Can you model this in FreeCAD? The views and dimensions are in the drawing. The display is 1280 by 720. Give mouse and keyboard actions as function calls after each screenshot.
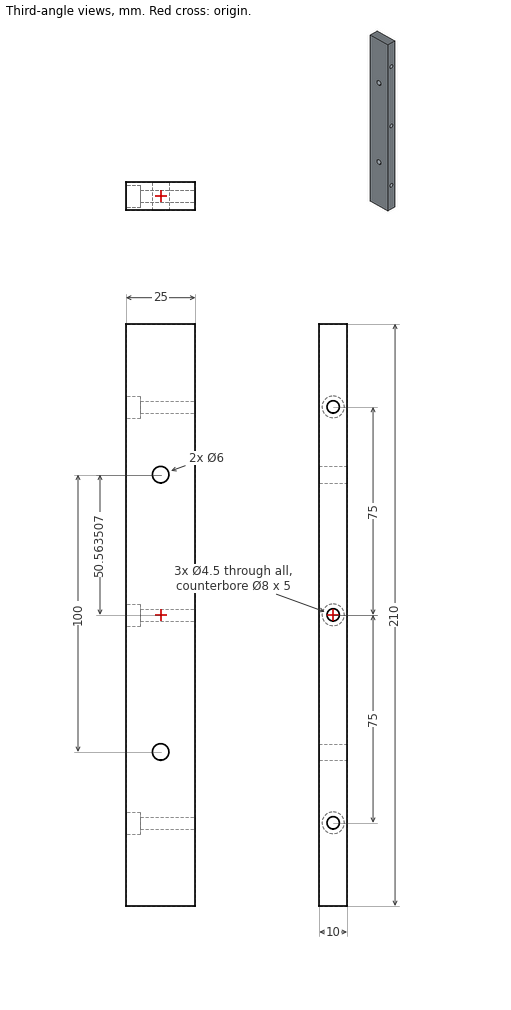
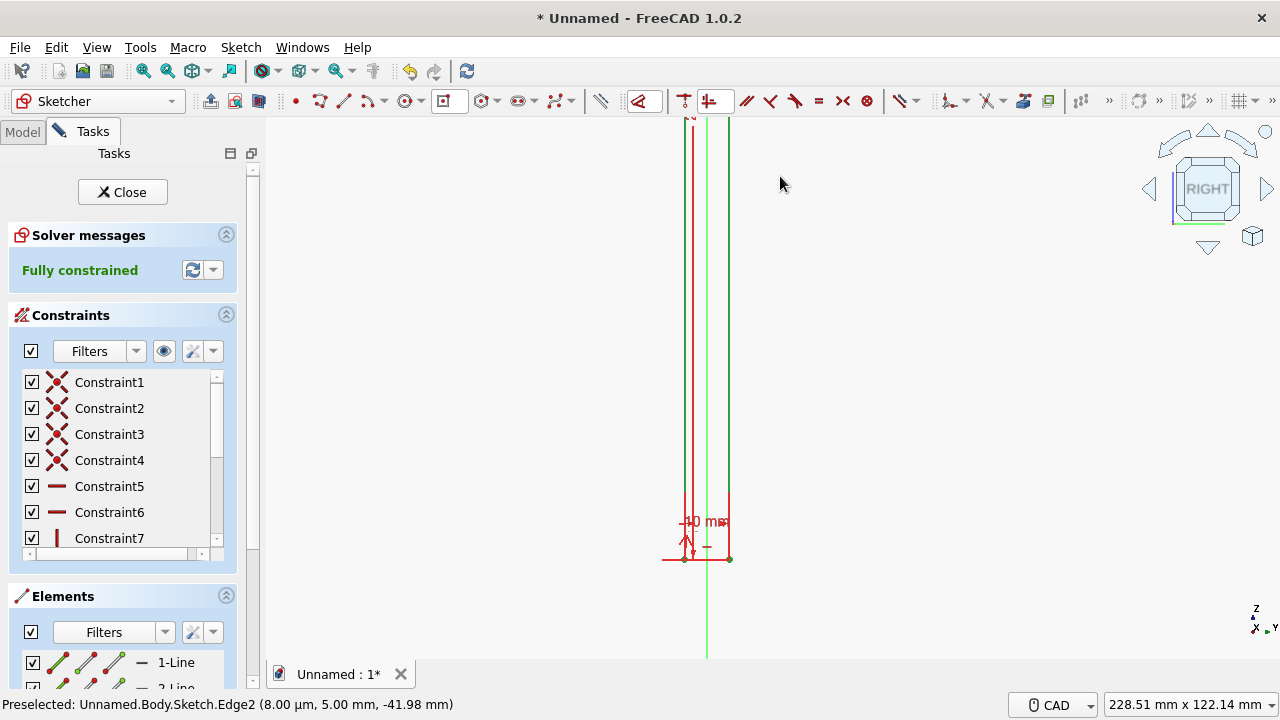
click(123, 192)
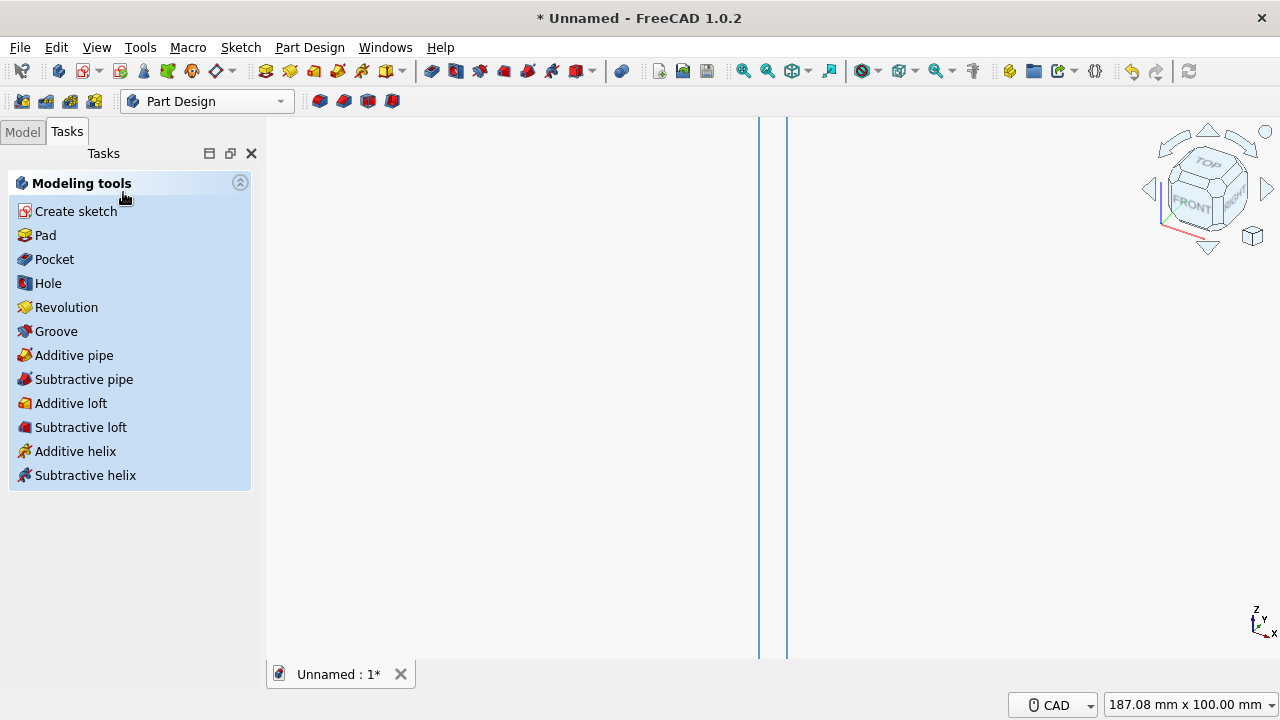
click(266, 72)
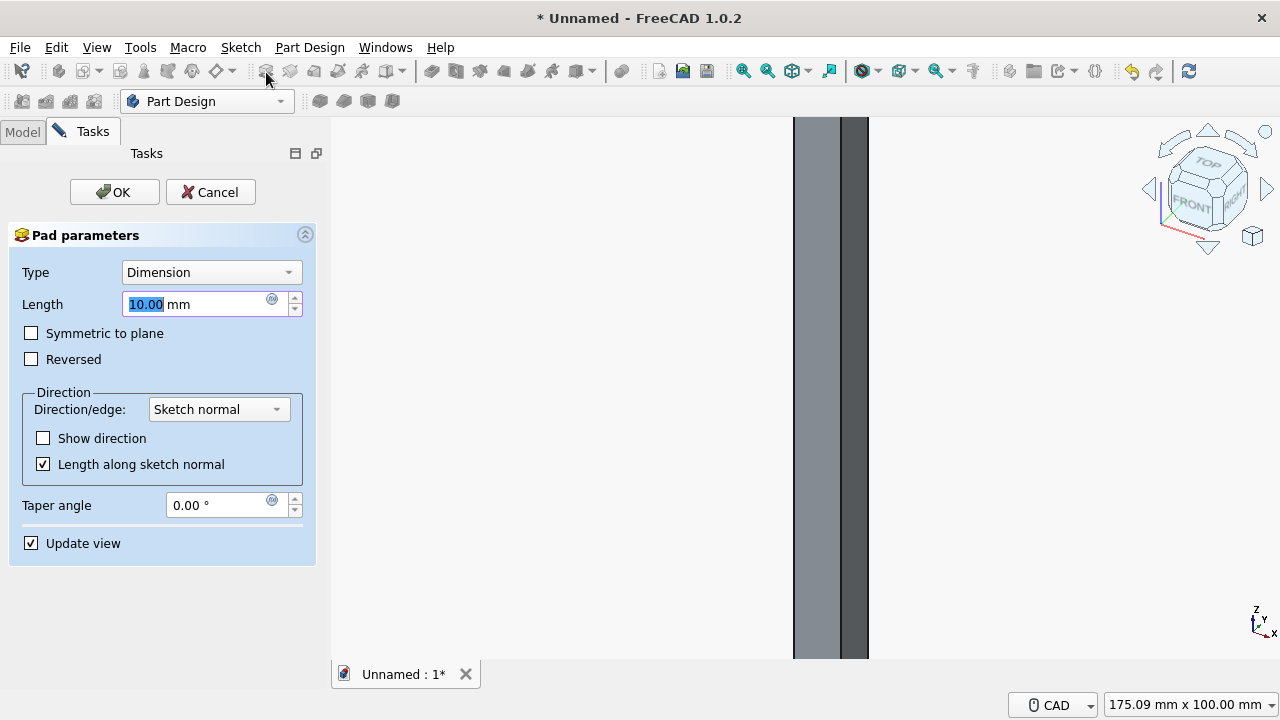
text(25)
key(Tab)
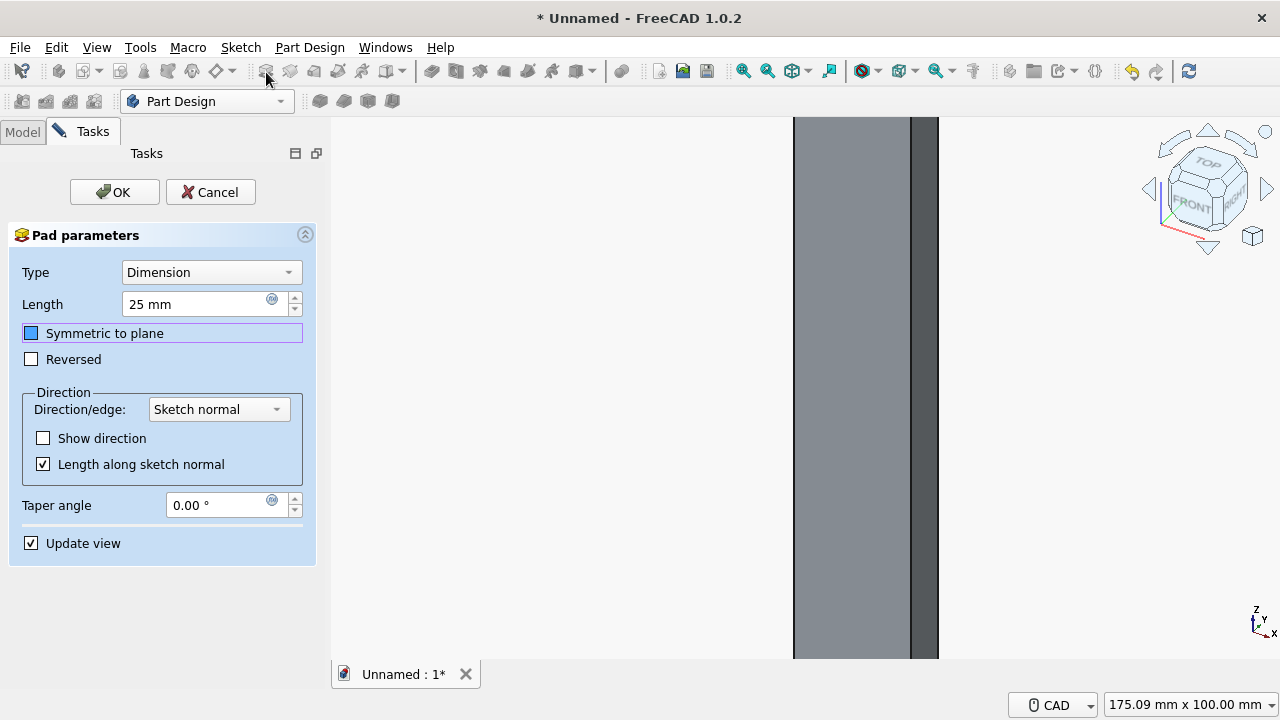
click(30, 333)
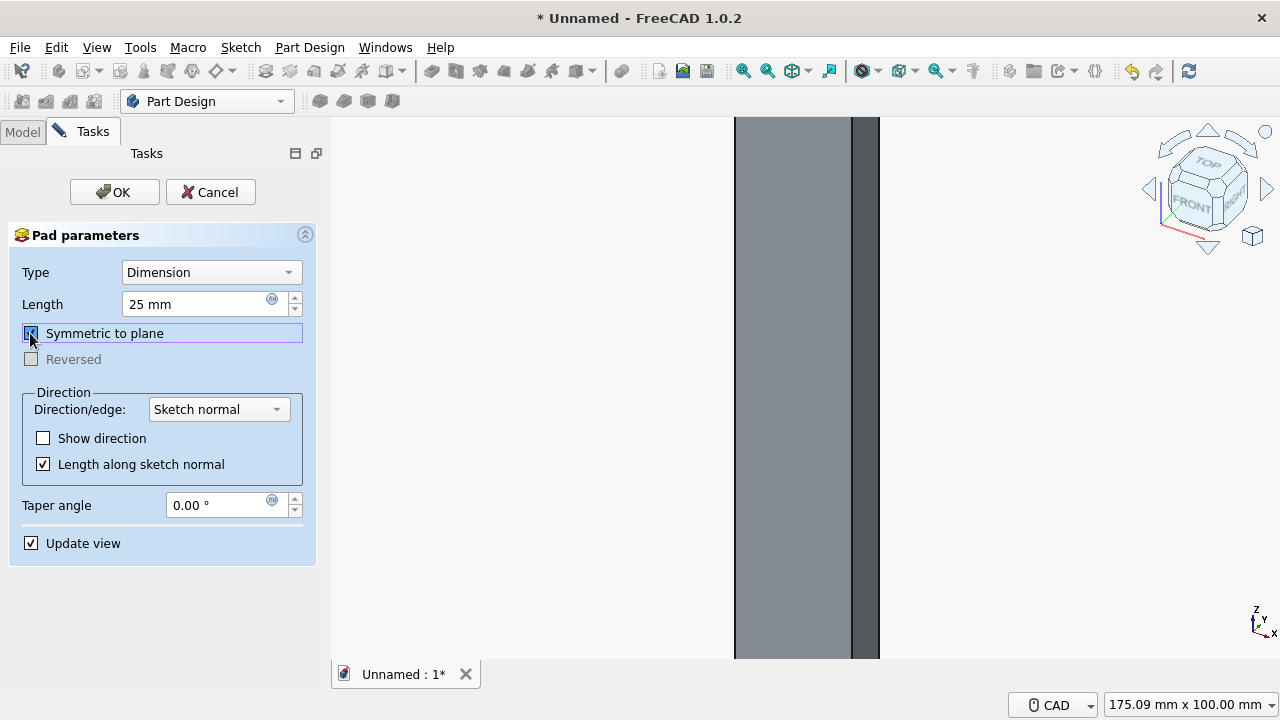
click(115, 192)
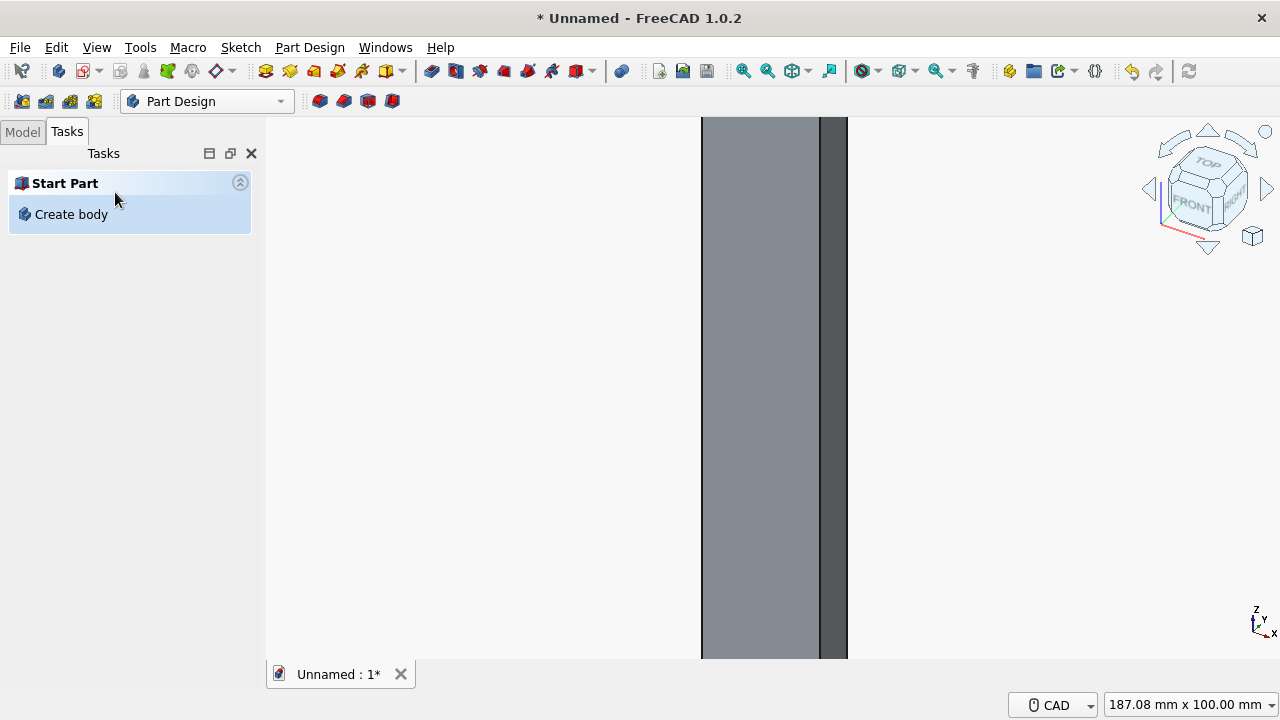
click(744, 72)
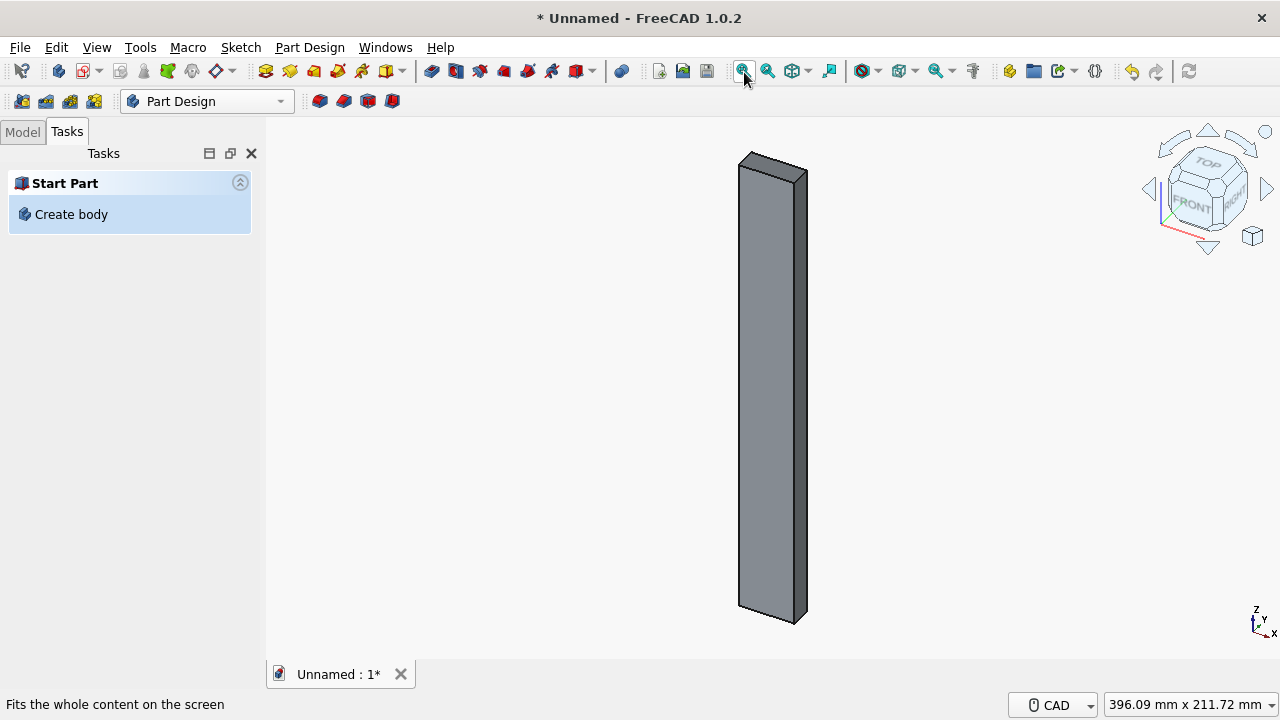
key(6)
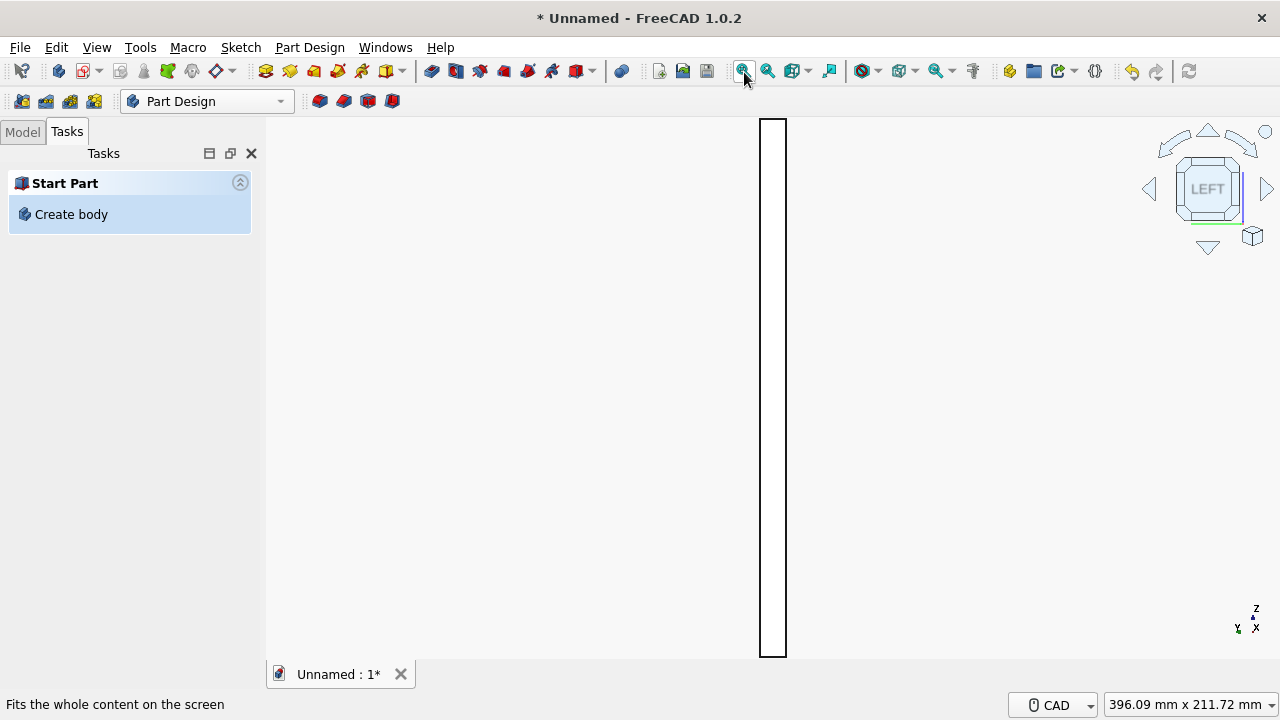
click(773, 617)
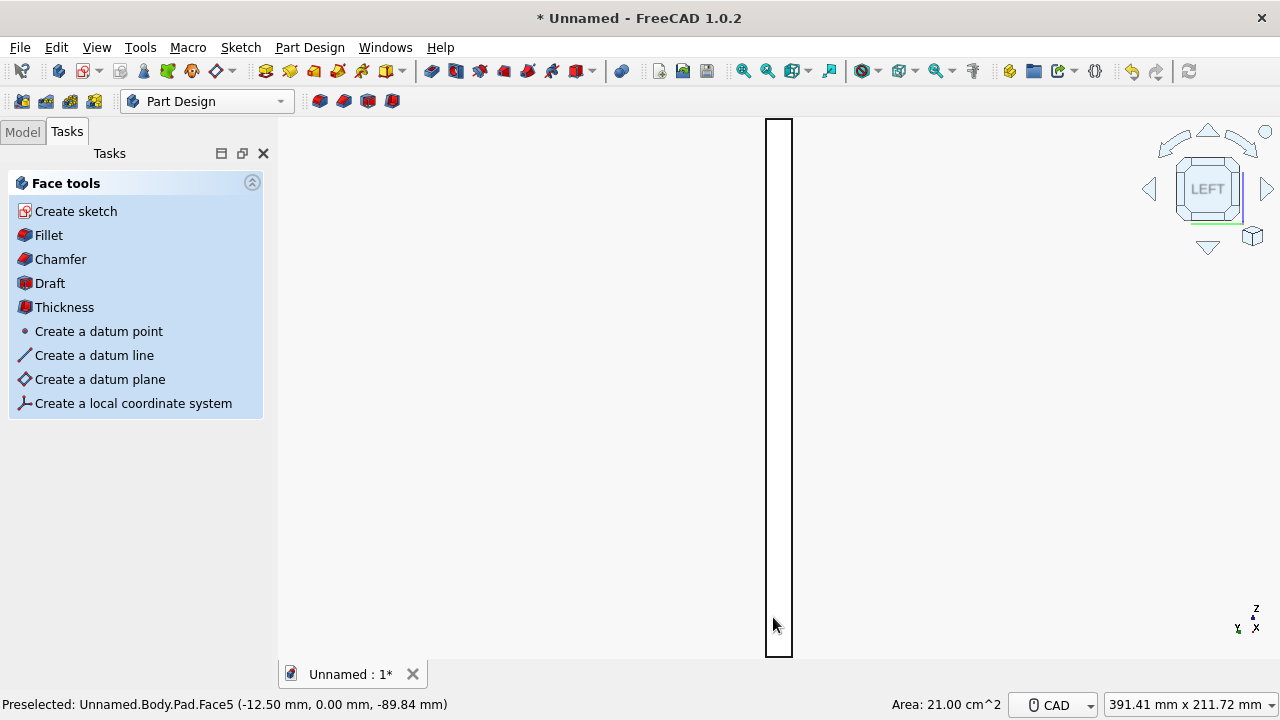
click(84, 72)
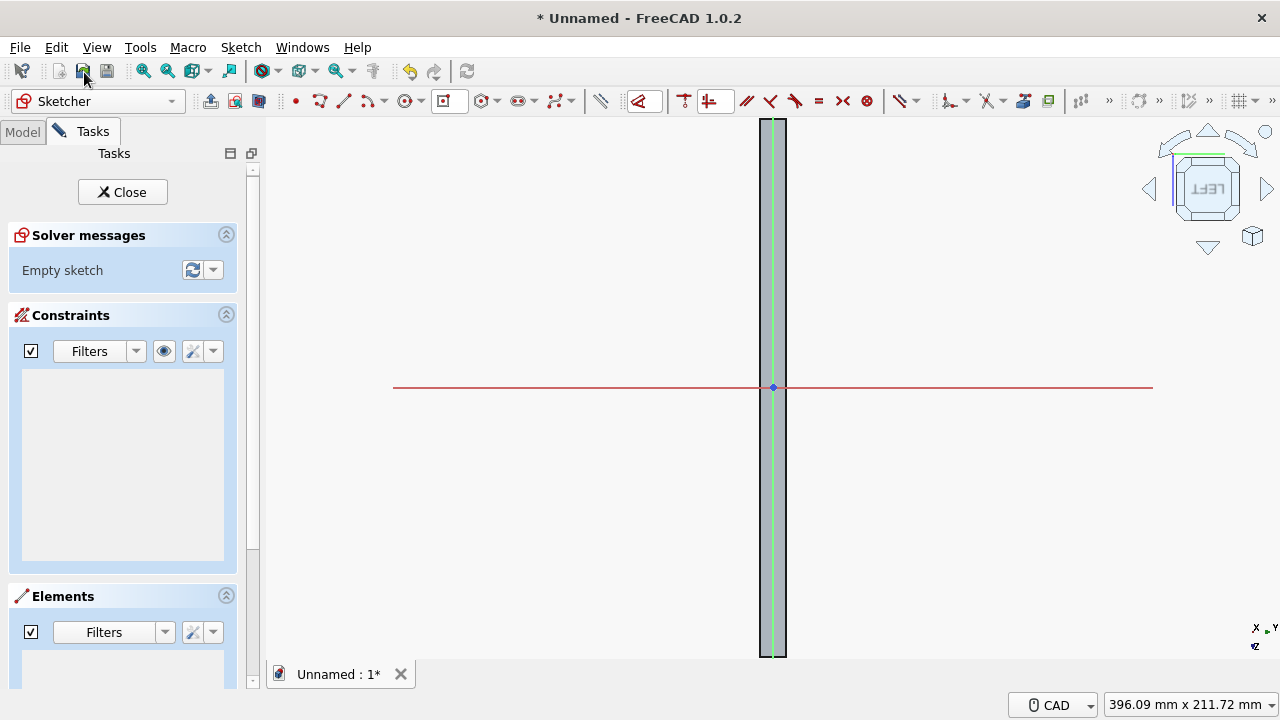
click(406, 102)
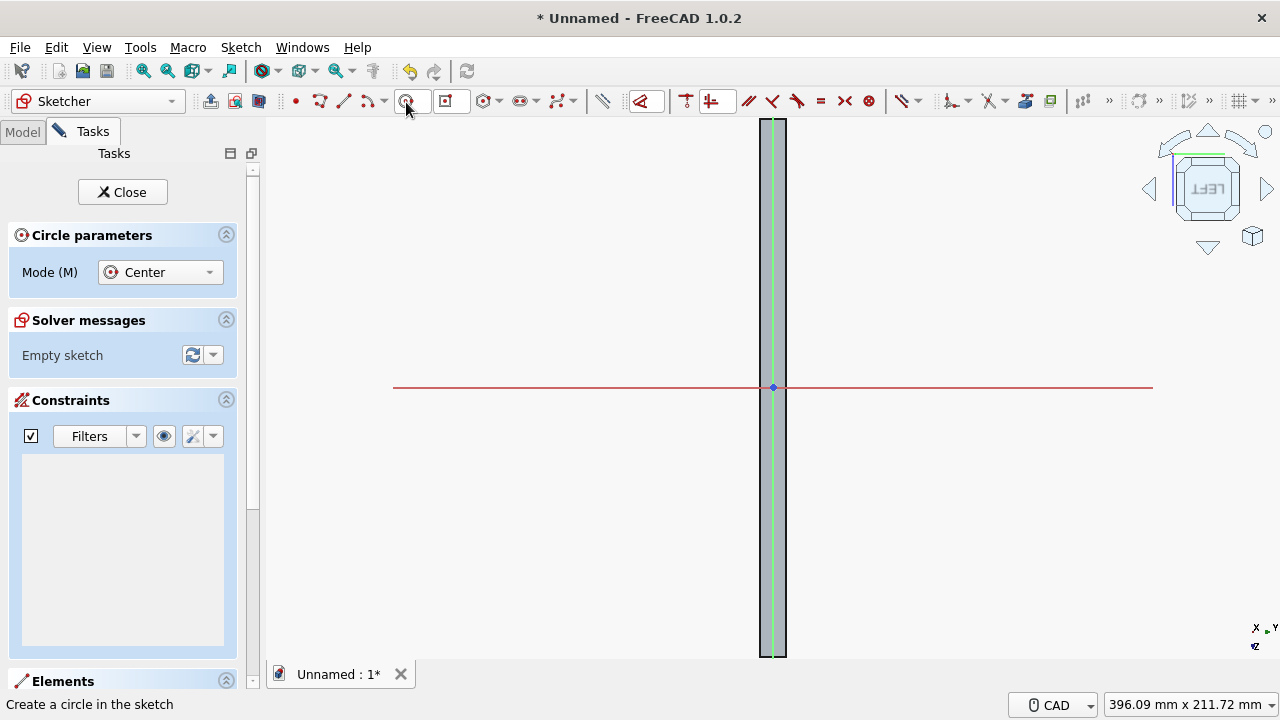
scroll(773, 388, up, 7)